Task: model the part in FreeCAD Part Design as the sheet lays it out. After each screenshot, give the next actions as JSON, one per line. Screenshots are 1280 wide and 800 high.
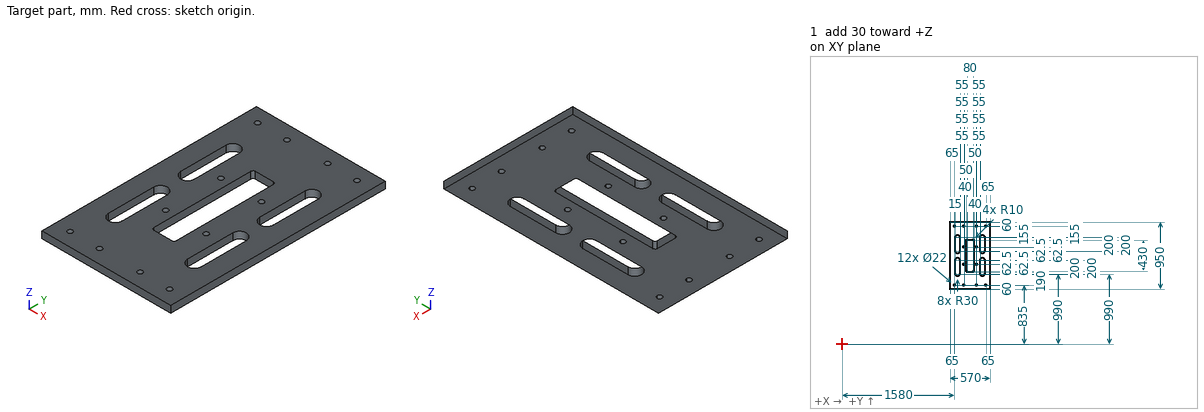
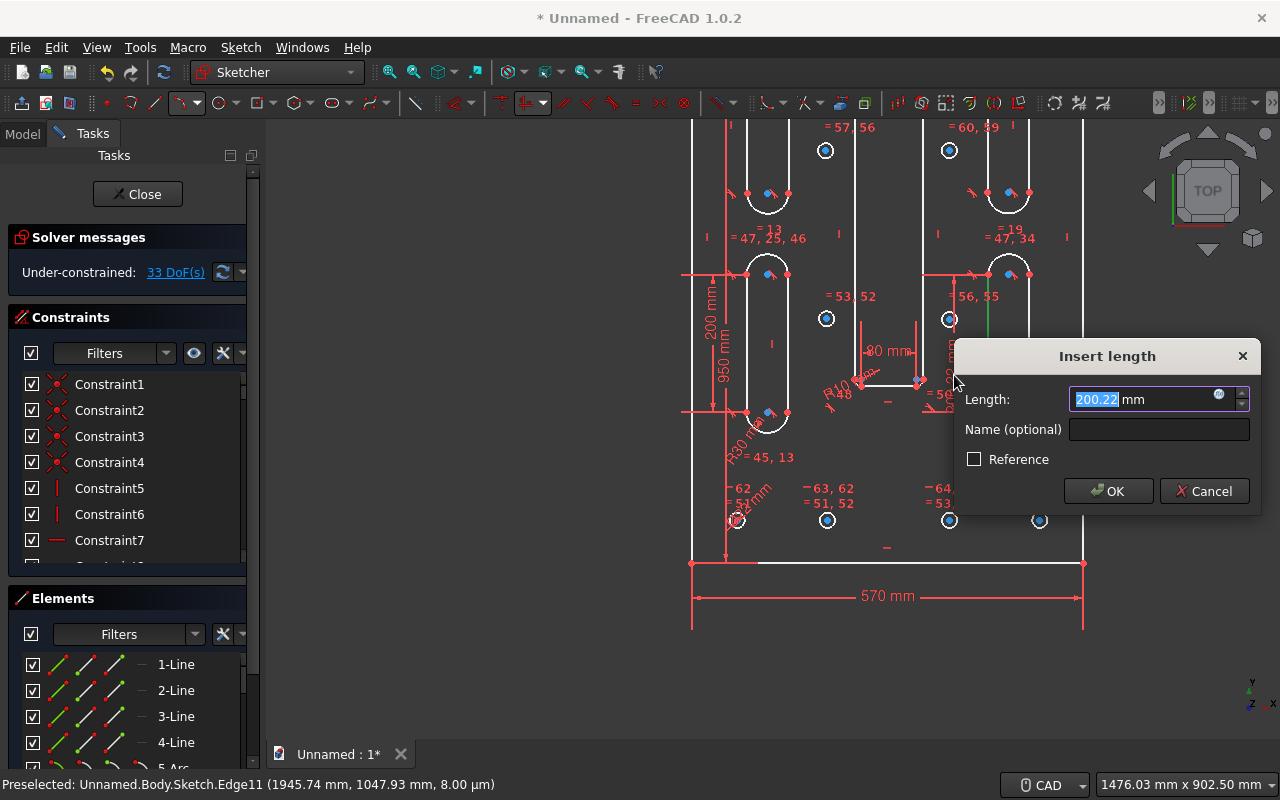
{"action": "type", "text": "200"}
{"action": "key", "text": "Return"}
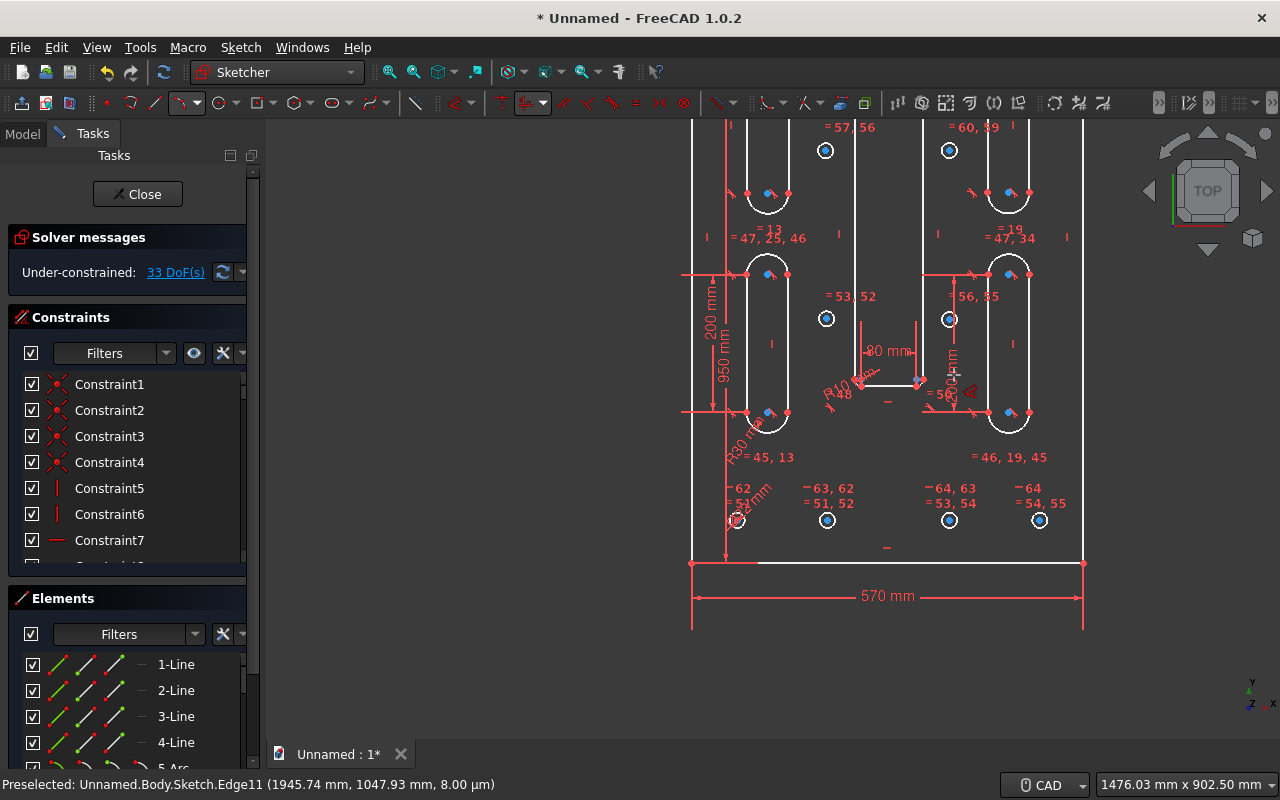
{"action": "left_click", "coordinate": [747, 152]}
{"action": "left_click", "coordinate": [713, 170]}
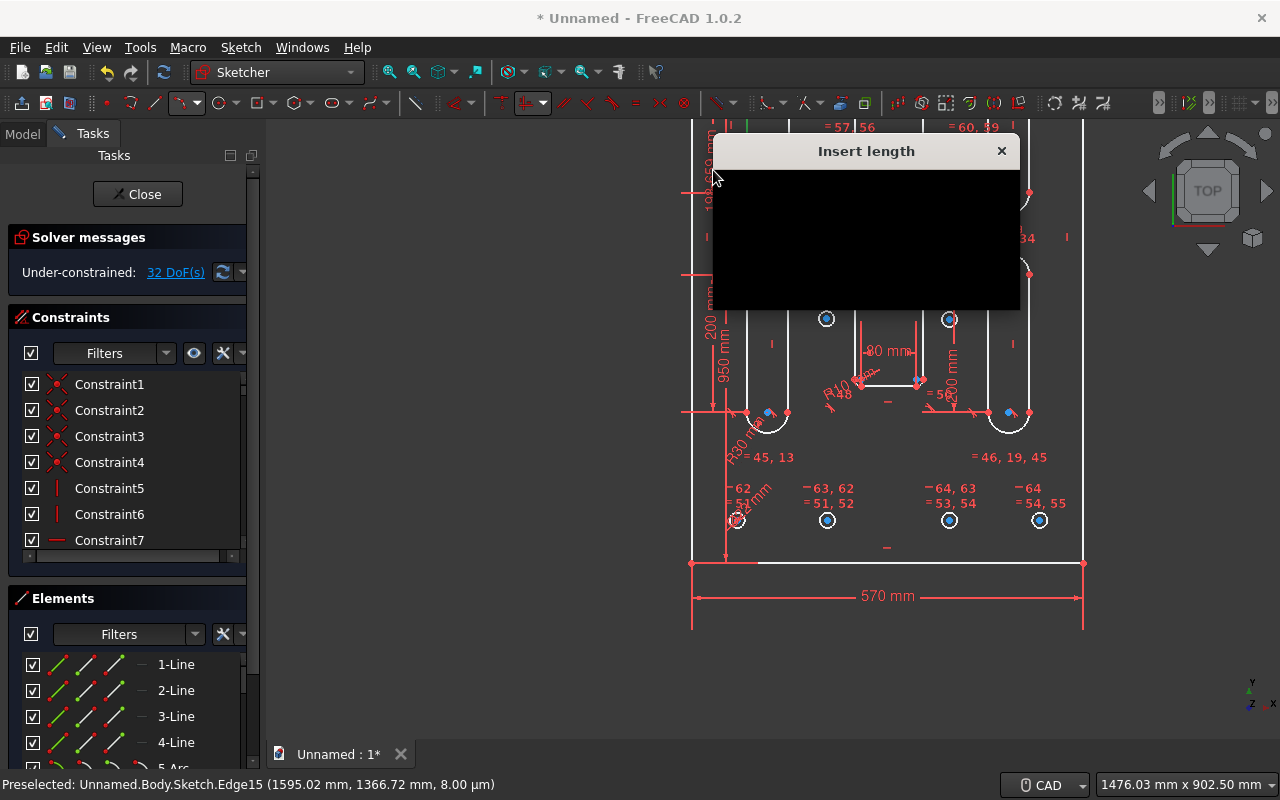
{"action": "type", "text": "200"}
{"action": "key", "text": "Return"}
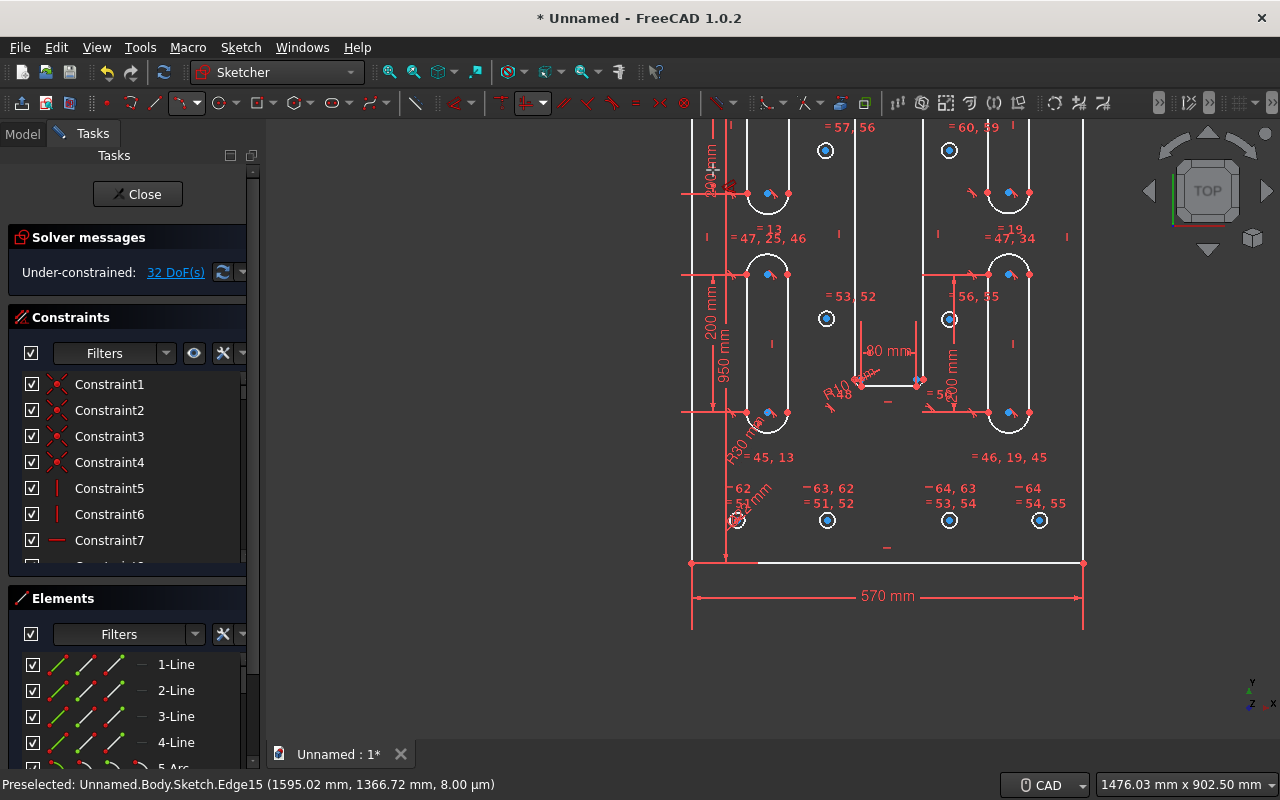
{"action": "left_click", "coordinate": [855, 292]}
{"action": "left_click", "coordinate": [889, 263]}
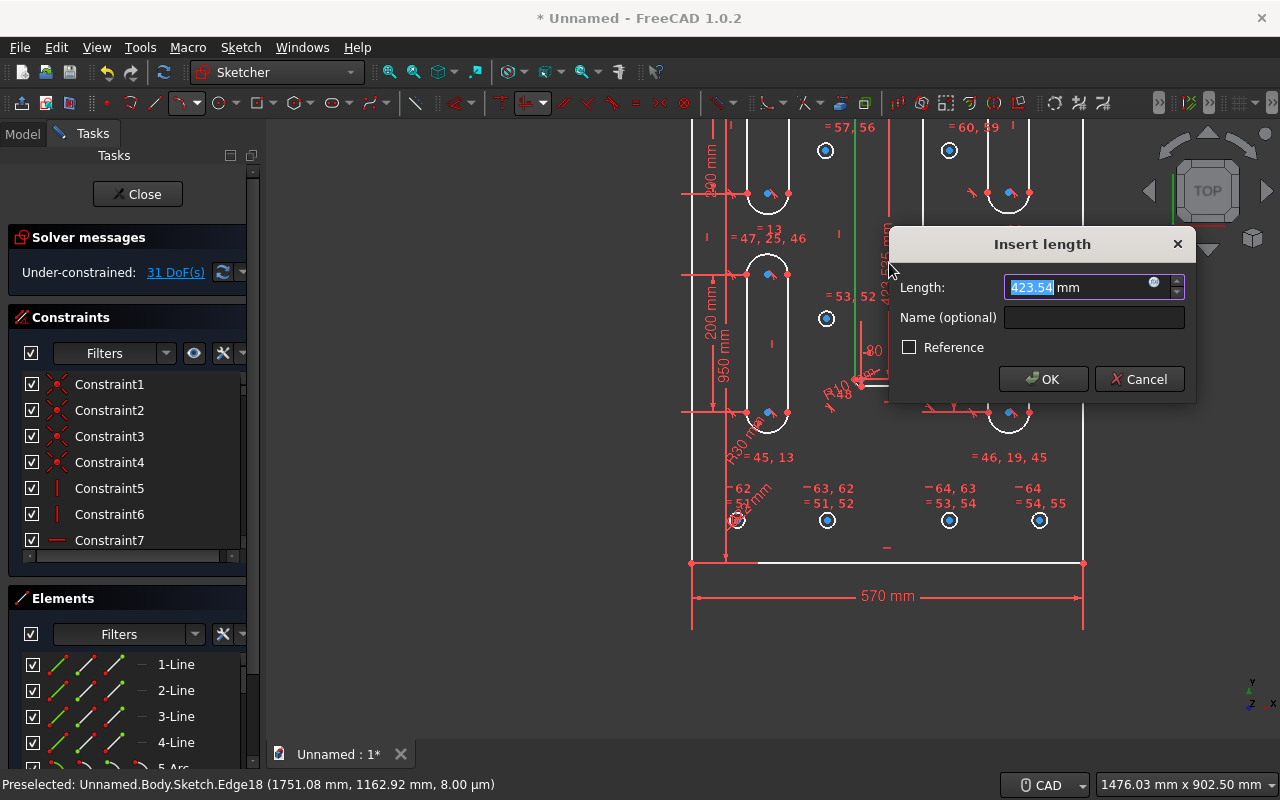
{"action": "type", "text": "430"}
{"action": "key", "text": "Return"}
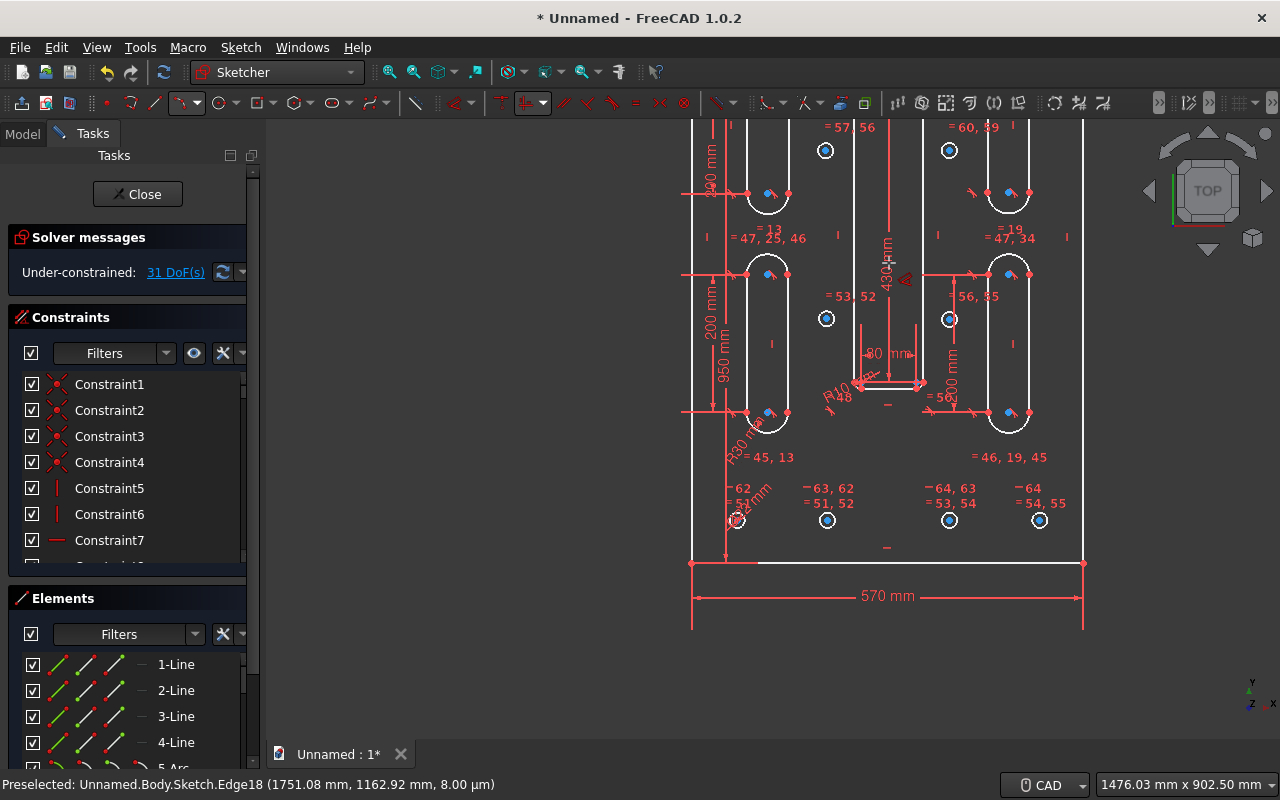
{"action": "left_click", "coordinate": [988, 152]}
{"action": "left_click", "coordinate": [954, 180]}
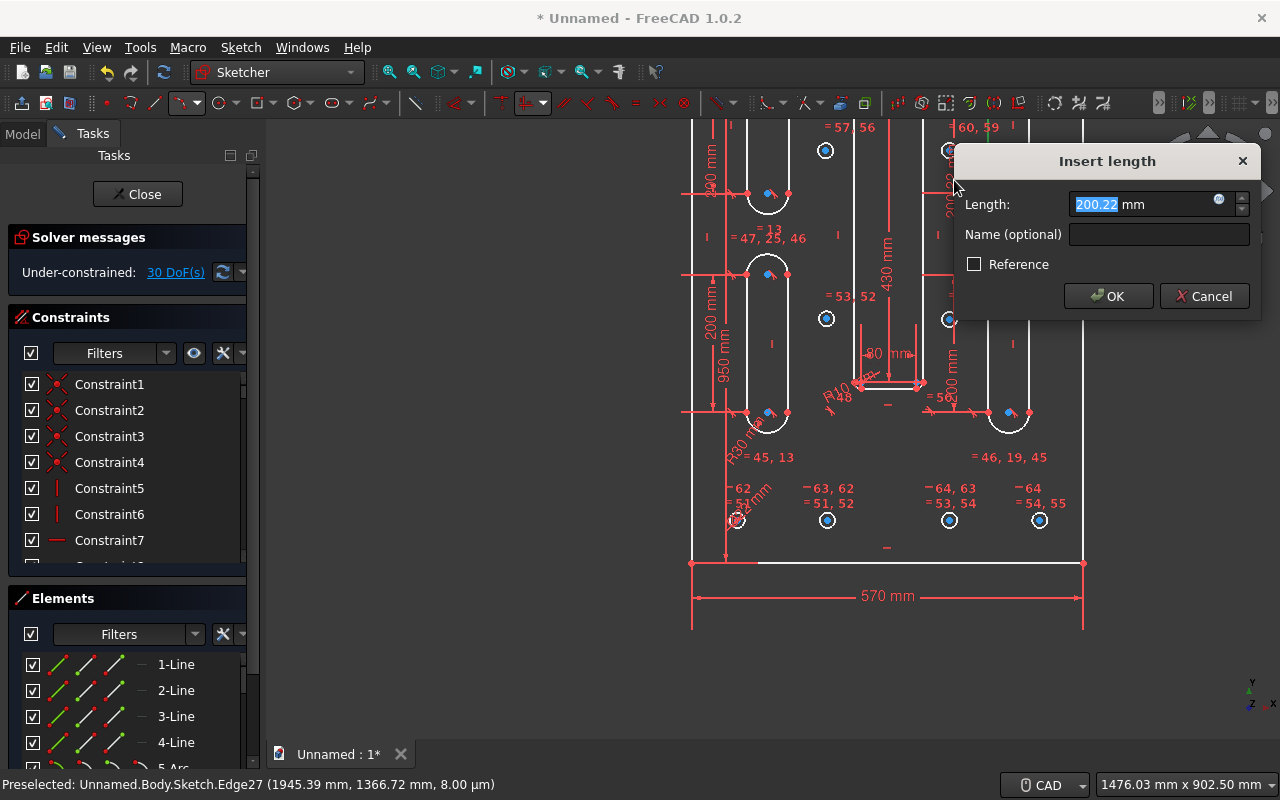
{"action": "type", "text": "200"}
{"action": "key", "text": "Return"}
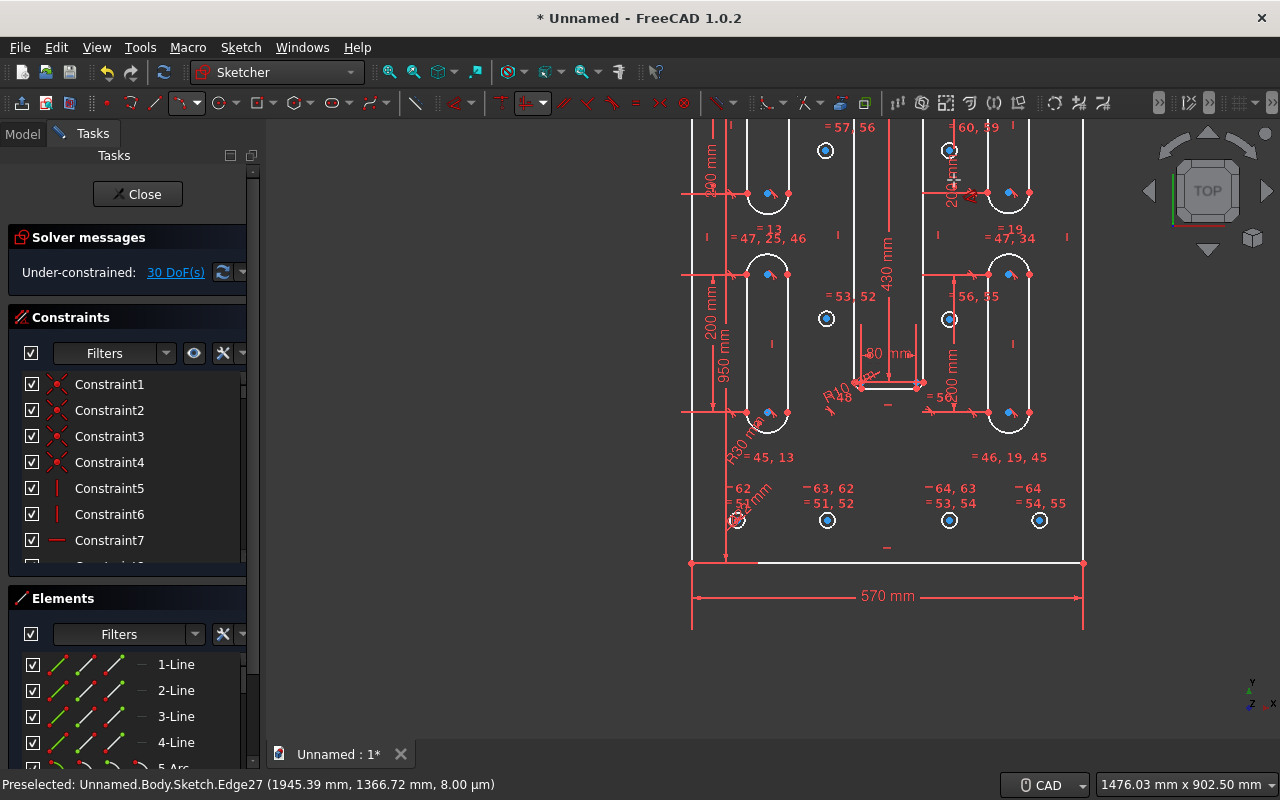
{"action": "left_click", "coordinate": [737, 520]}
{"action": "left_click", "coordinate": [771, 616]}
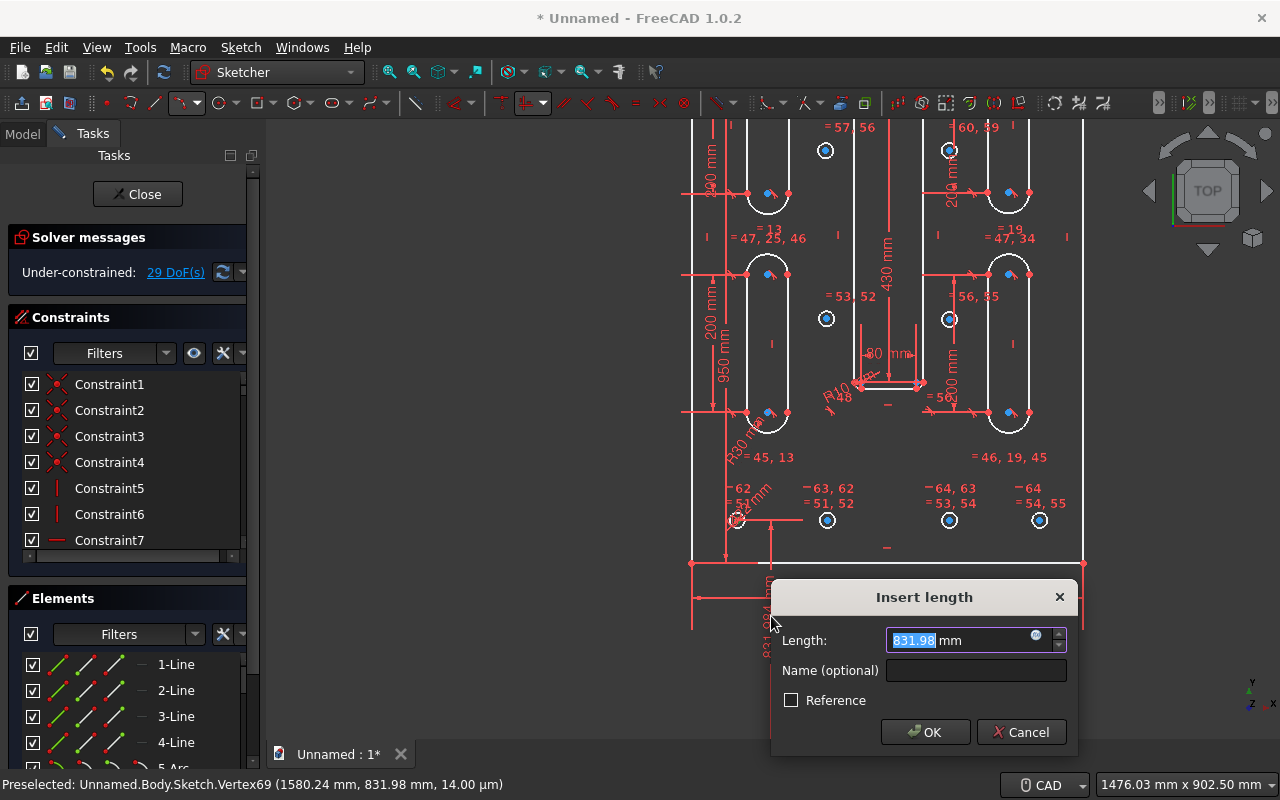
{"action": "type", "text": "835"}
{"action": "key", "text": "Return"}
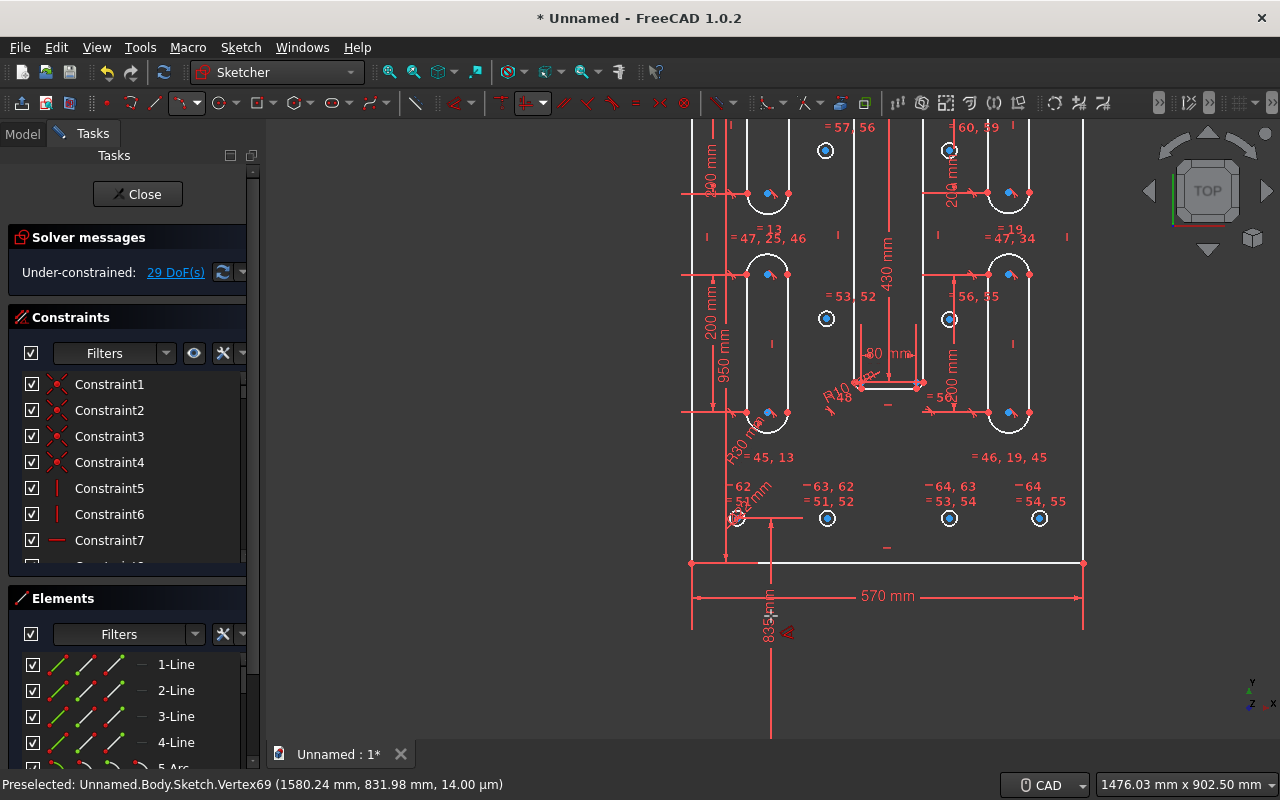
{"action": "left_click", "coordinate": [692, 563]}